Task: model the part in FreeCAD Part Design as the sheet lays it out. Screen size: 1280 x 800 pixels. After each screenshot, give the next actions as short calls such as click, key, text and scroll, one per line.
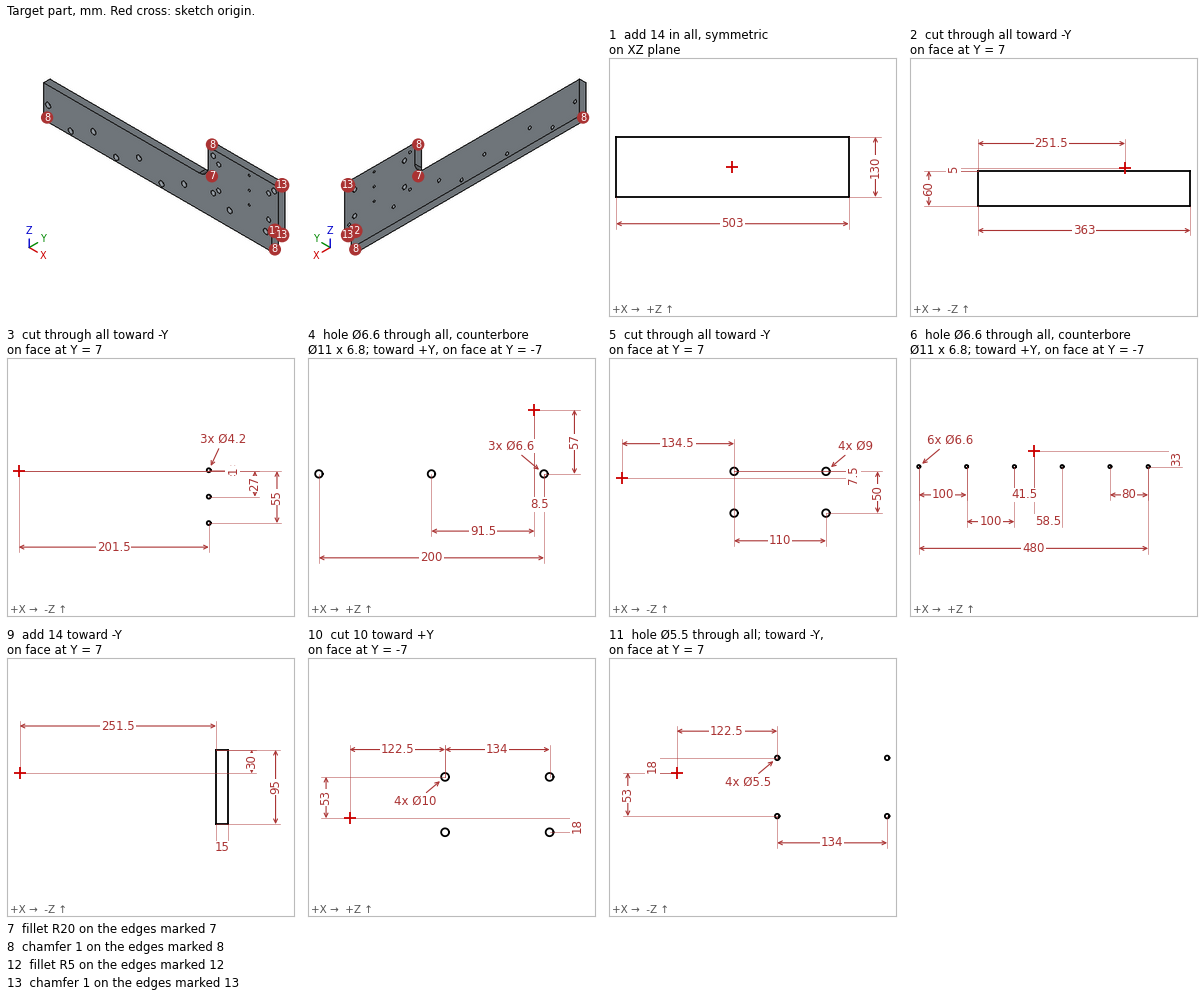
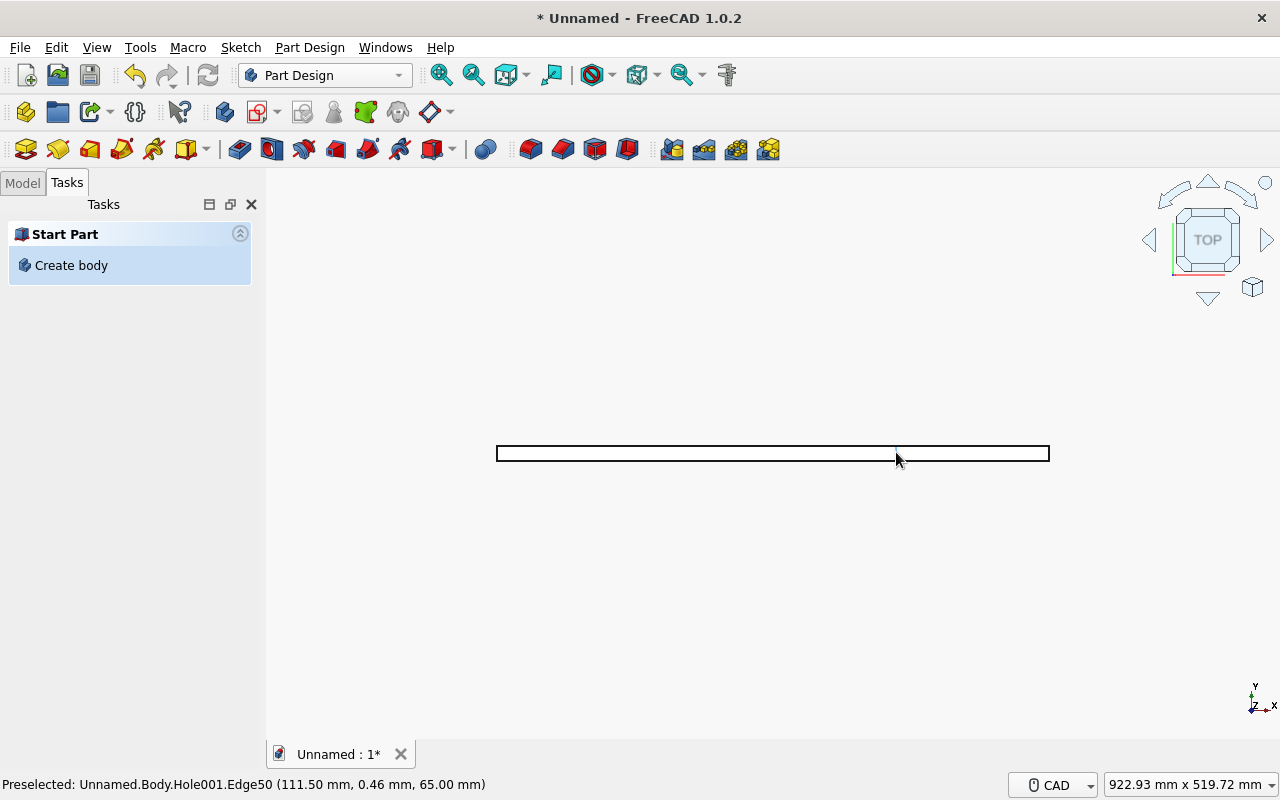
key(0)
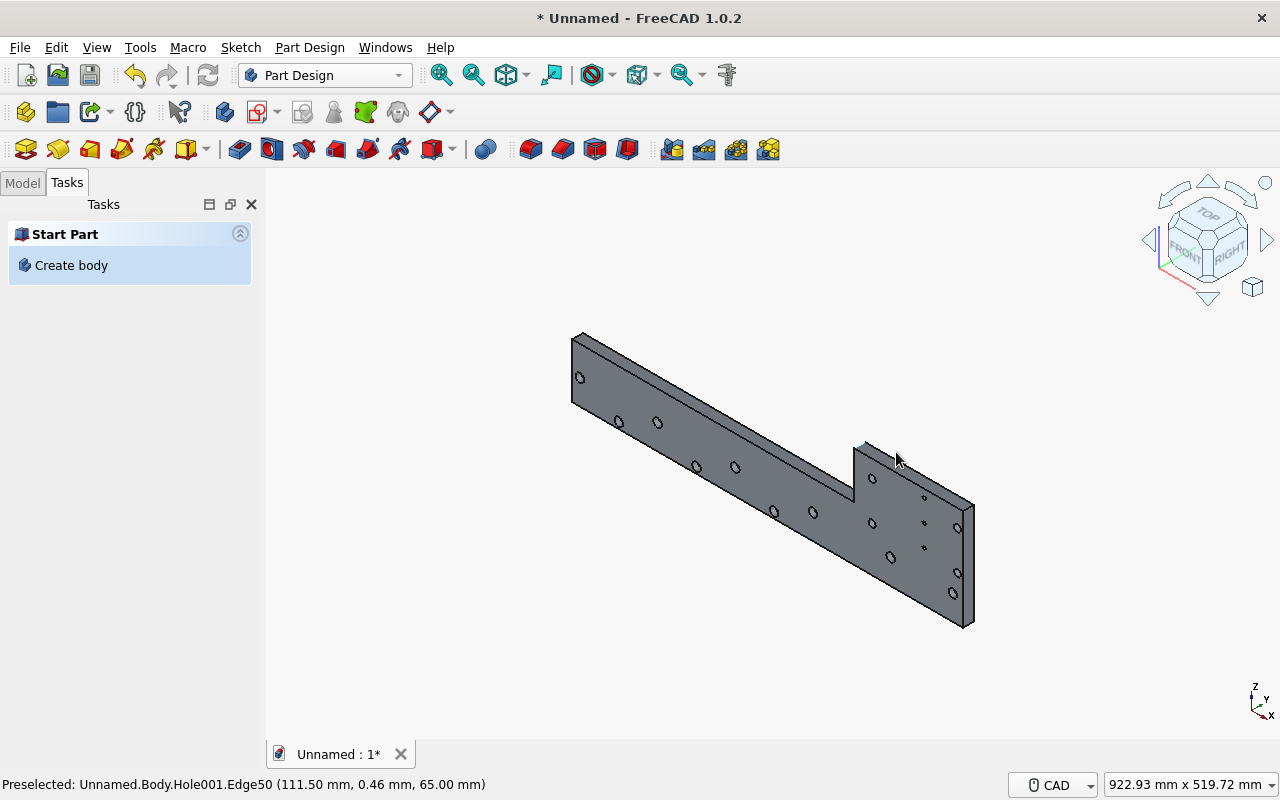
scroll(860, 498, up, 5)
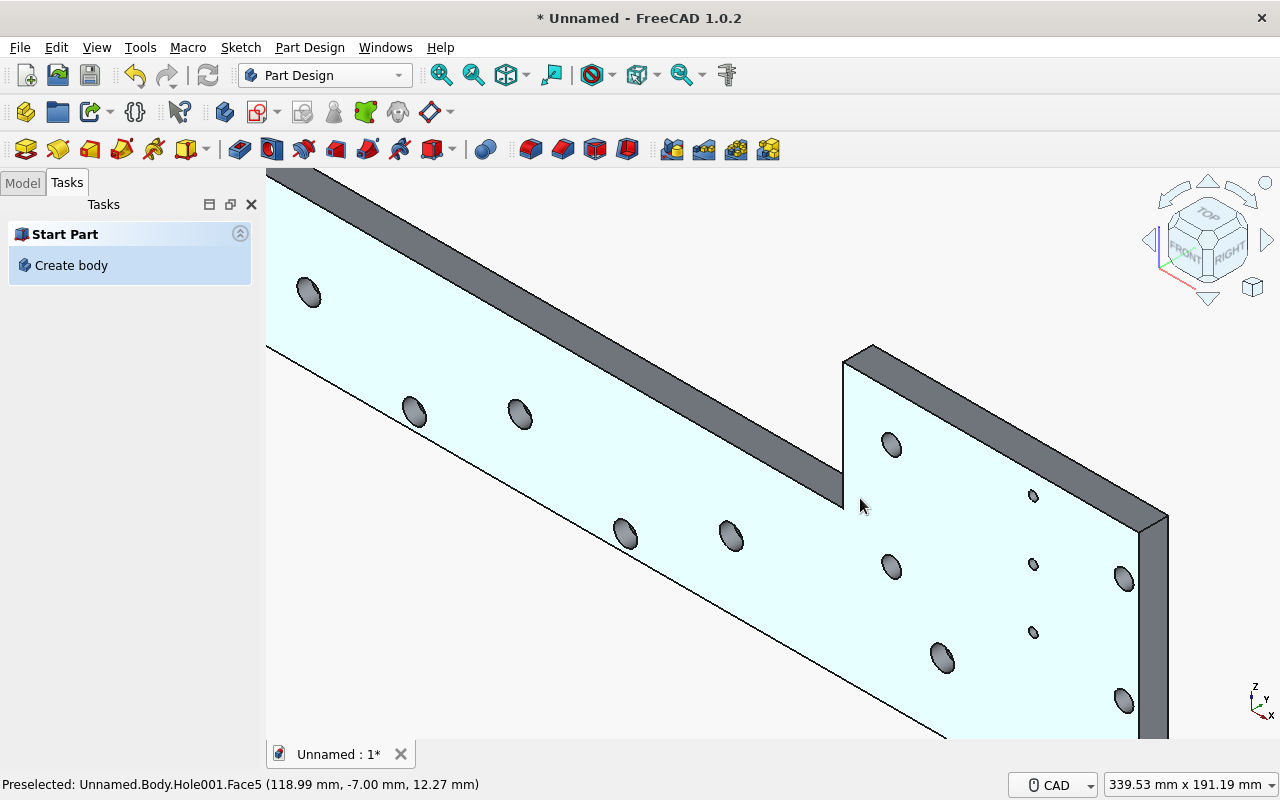
key(v)
key(f)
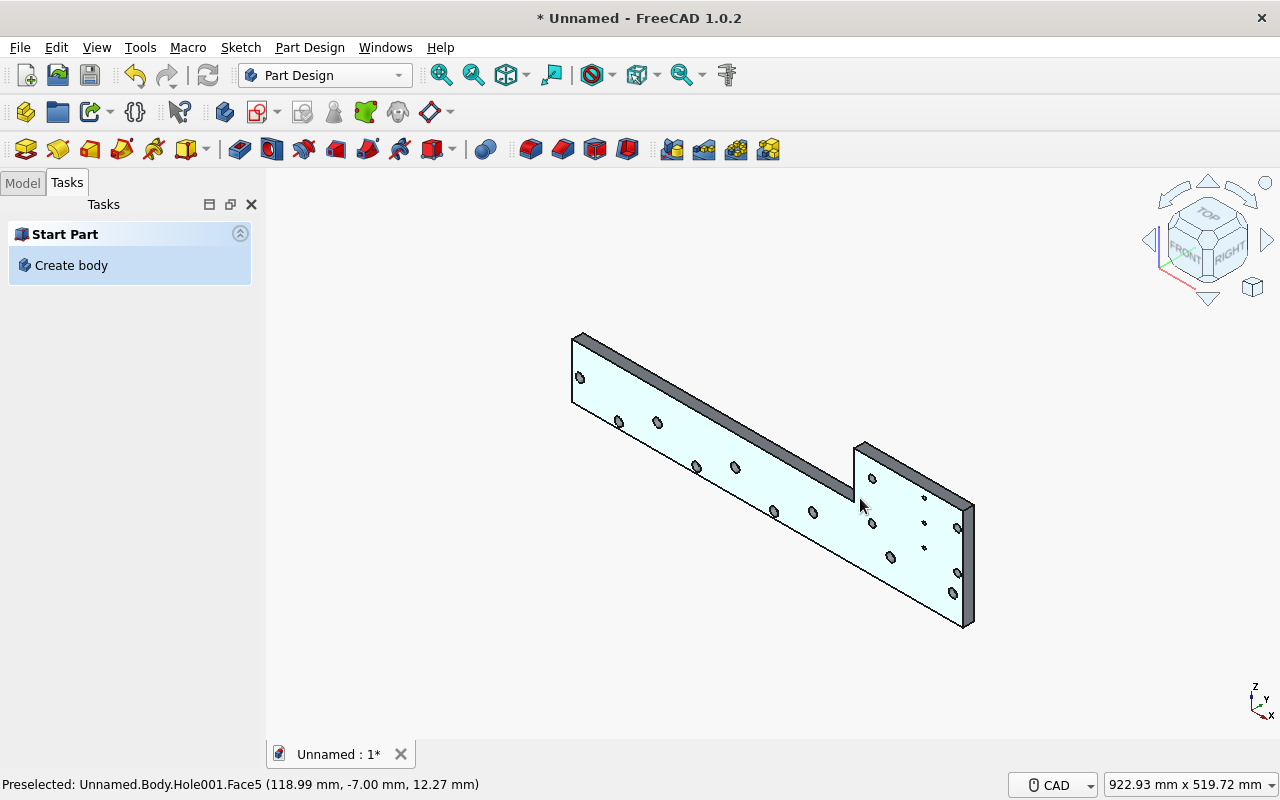
key(1)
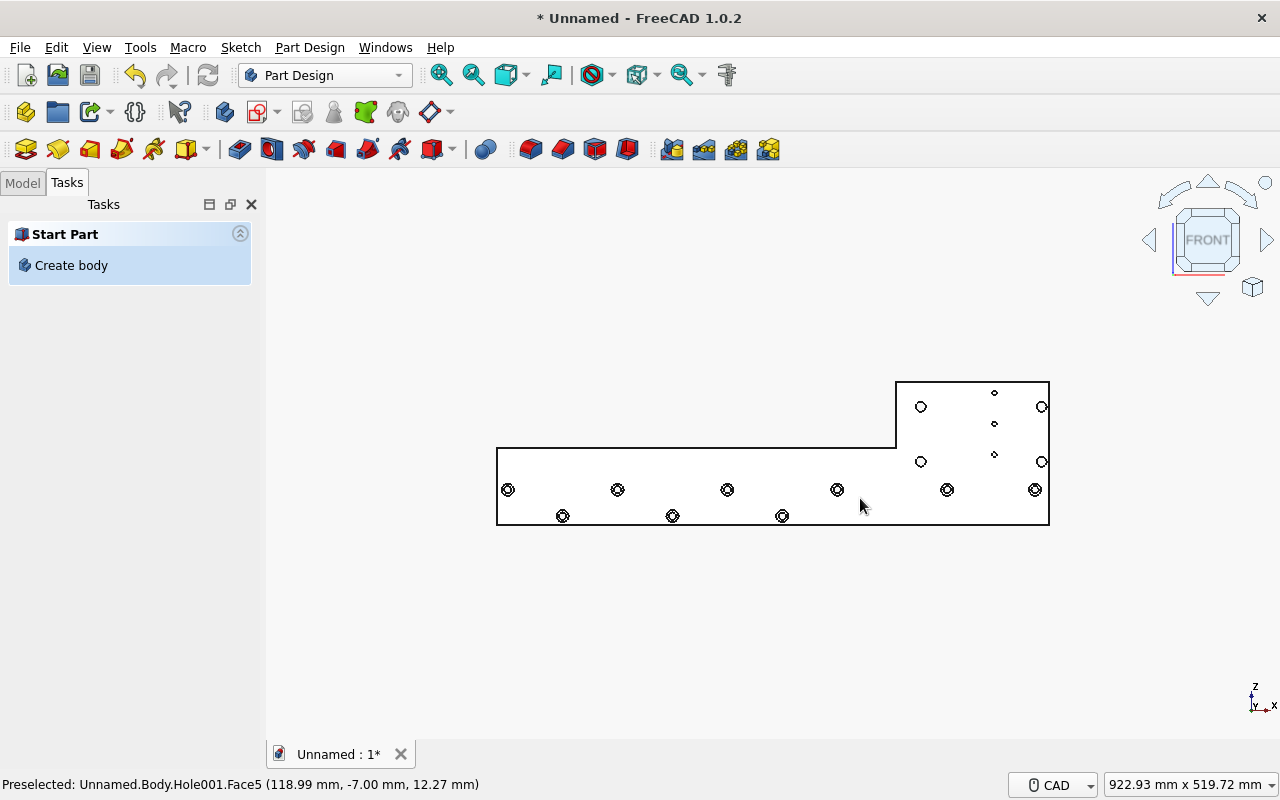
scroll(896, 447, up, 5)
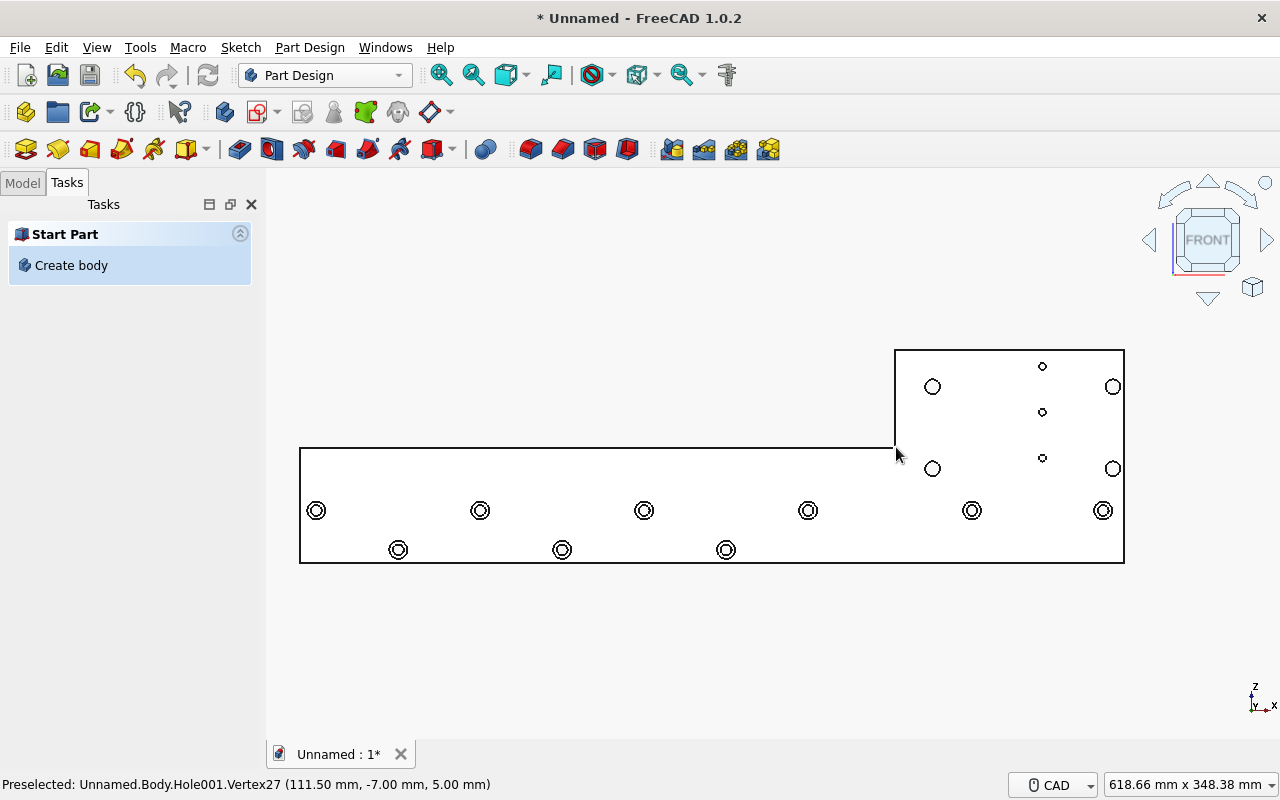
click(442, 76)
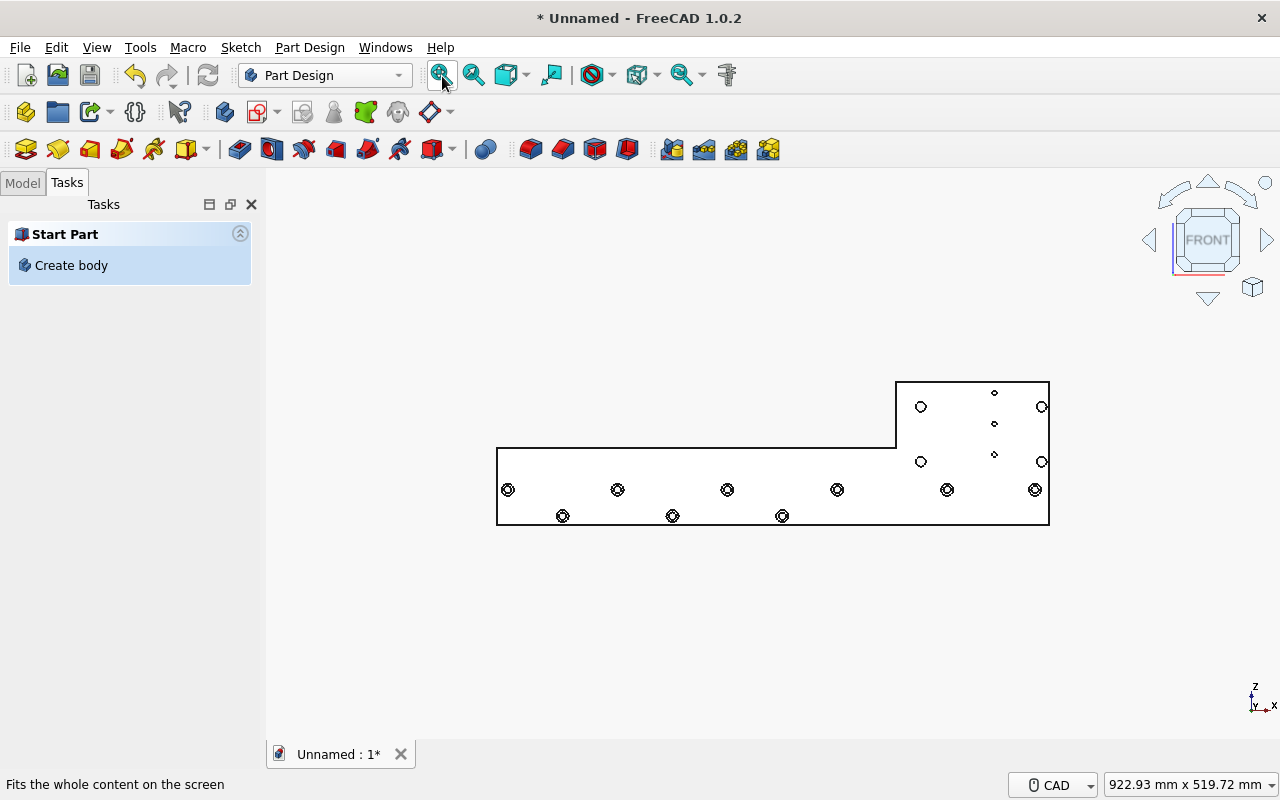
key(3)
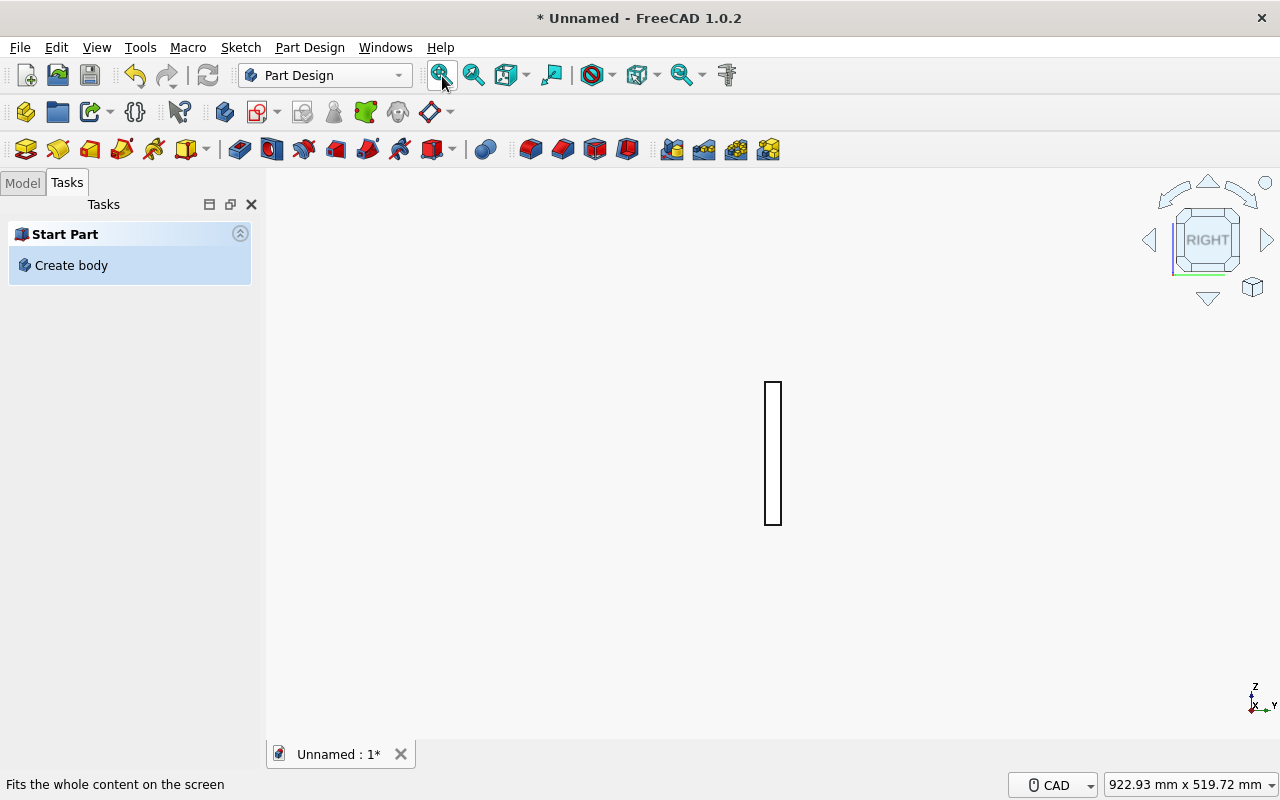
click(442, 76)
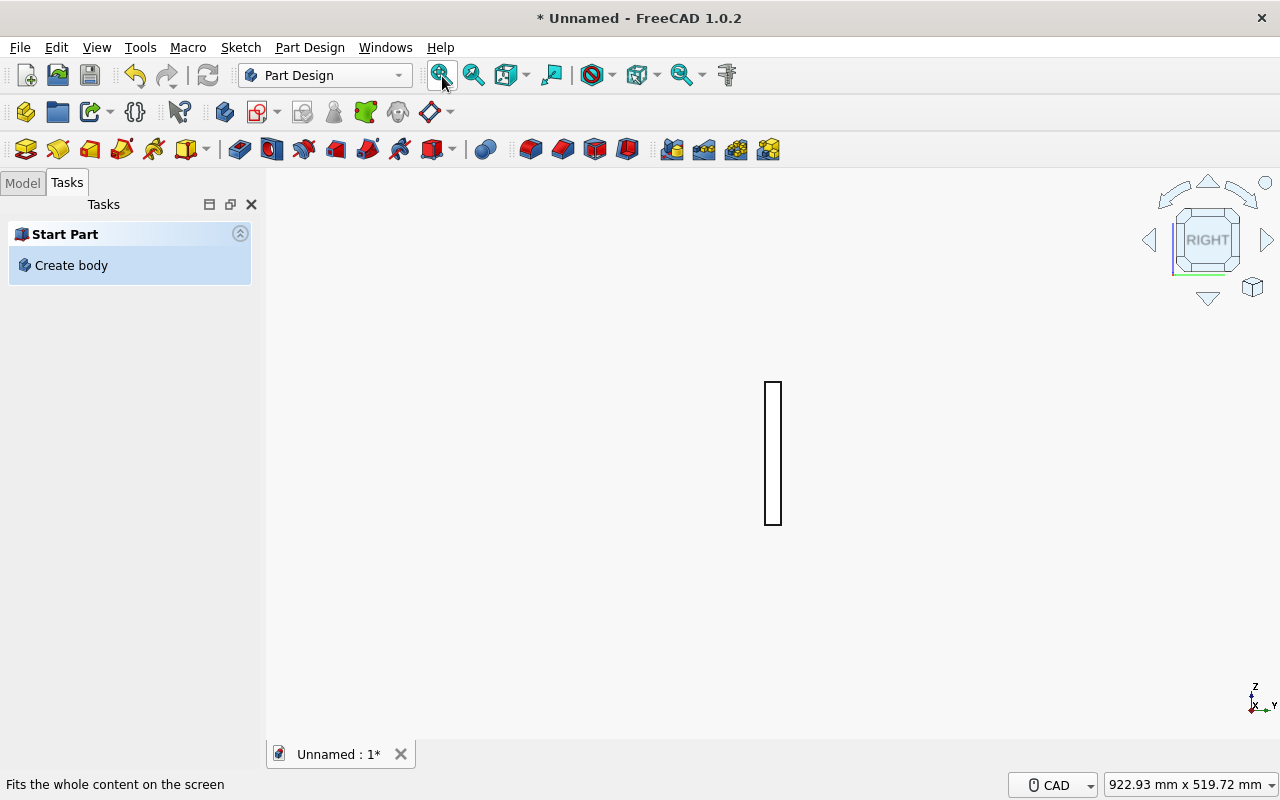
scroll(773, 447, up, 5)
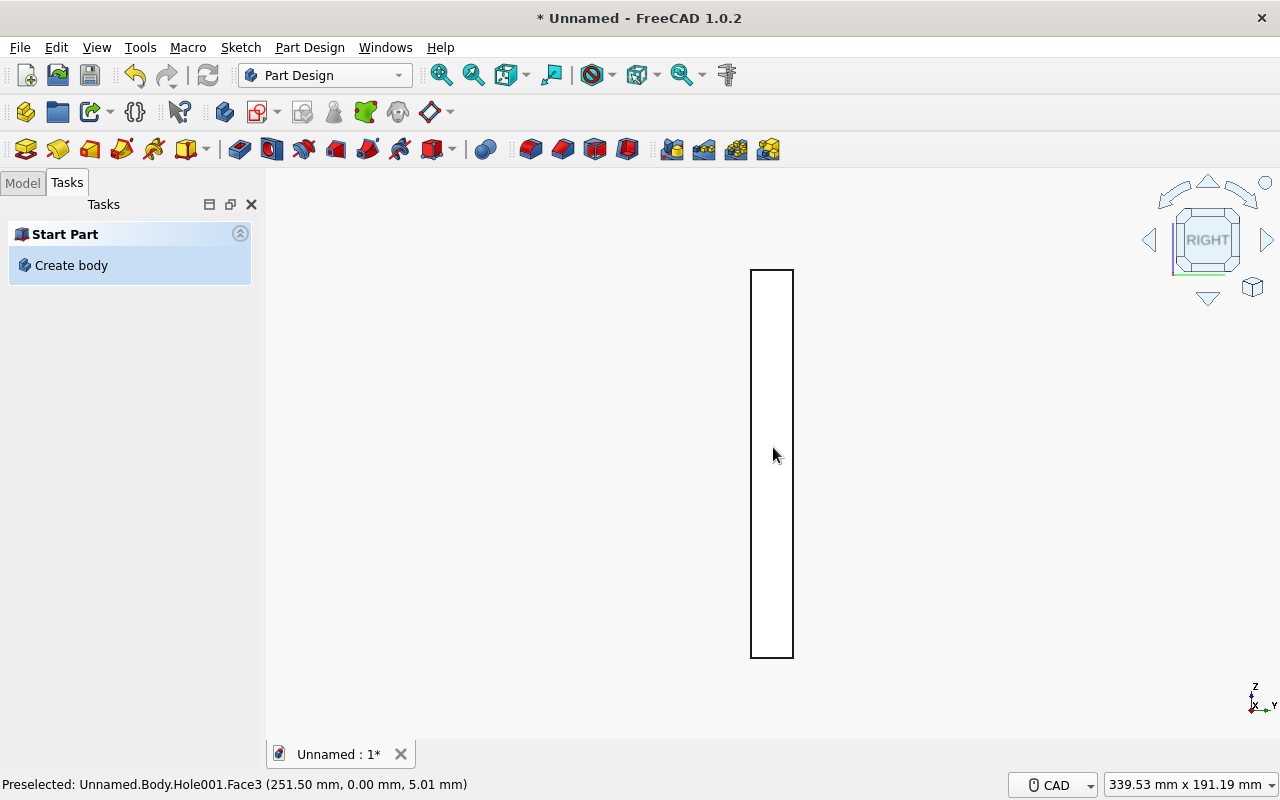
key(v)
key(f)